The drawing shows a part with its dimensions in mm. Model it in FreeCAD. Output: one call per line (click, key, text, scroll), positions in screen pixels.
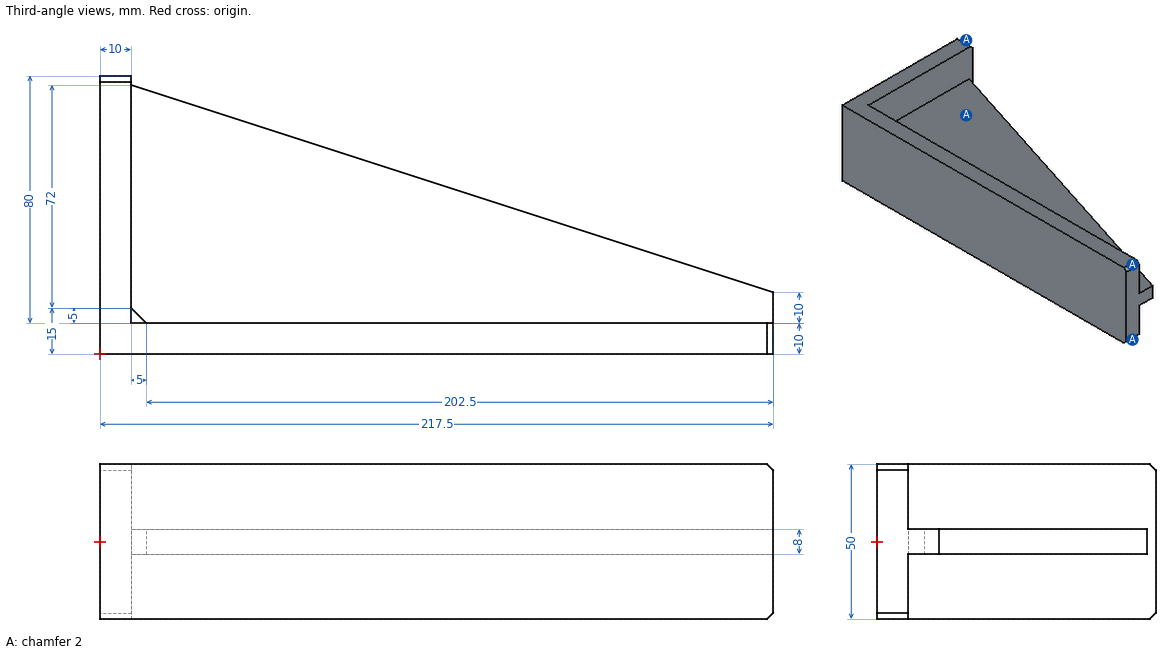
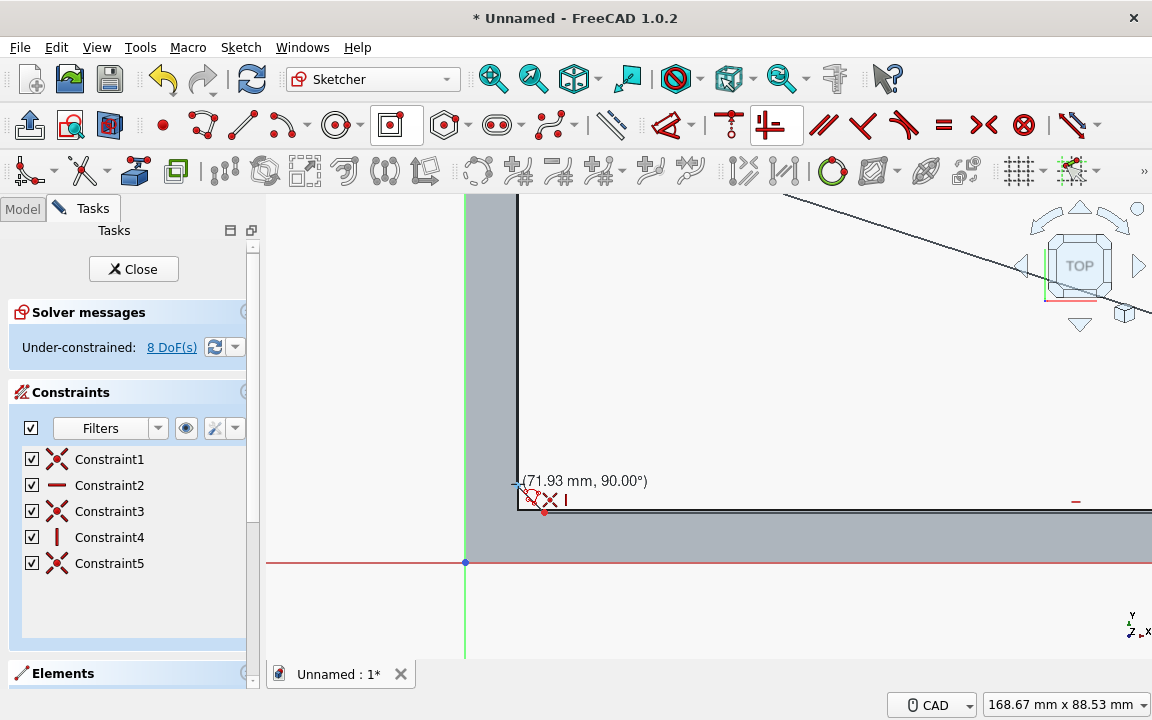
click(518, 486)
key(Escape)
key(Escape)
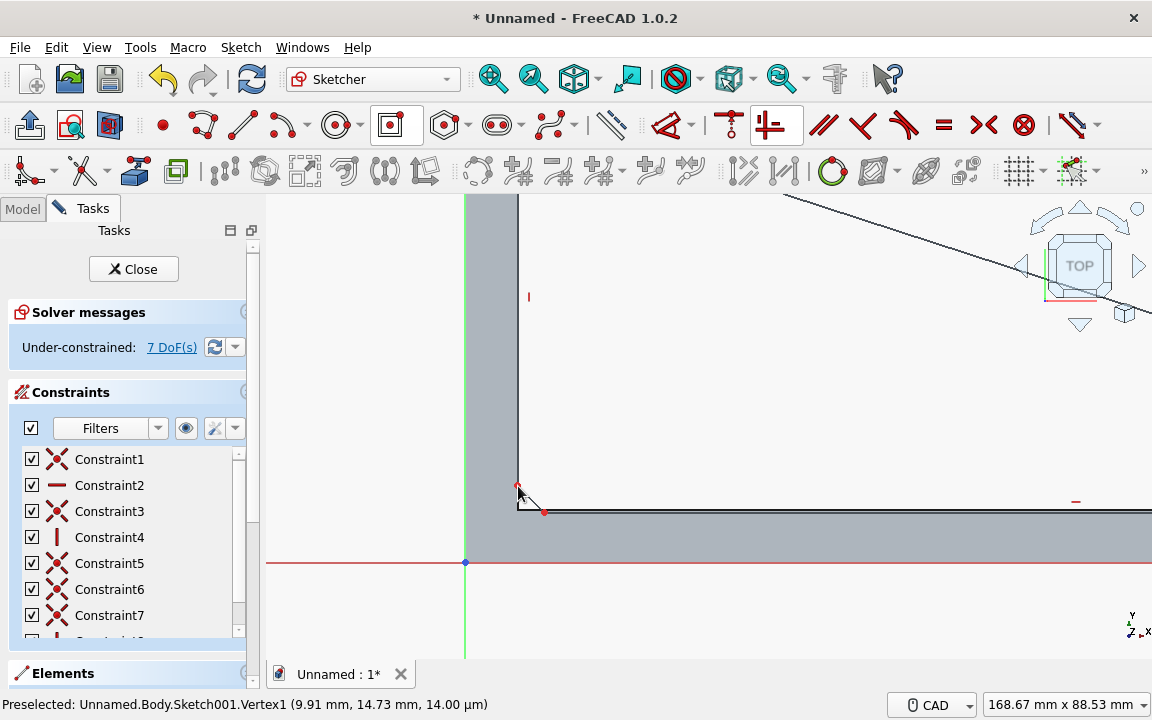
click(666, 126)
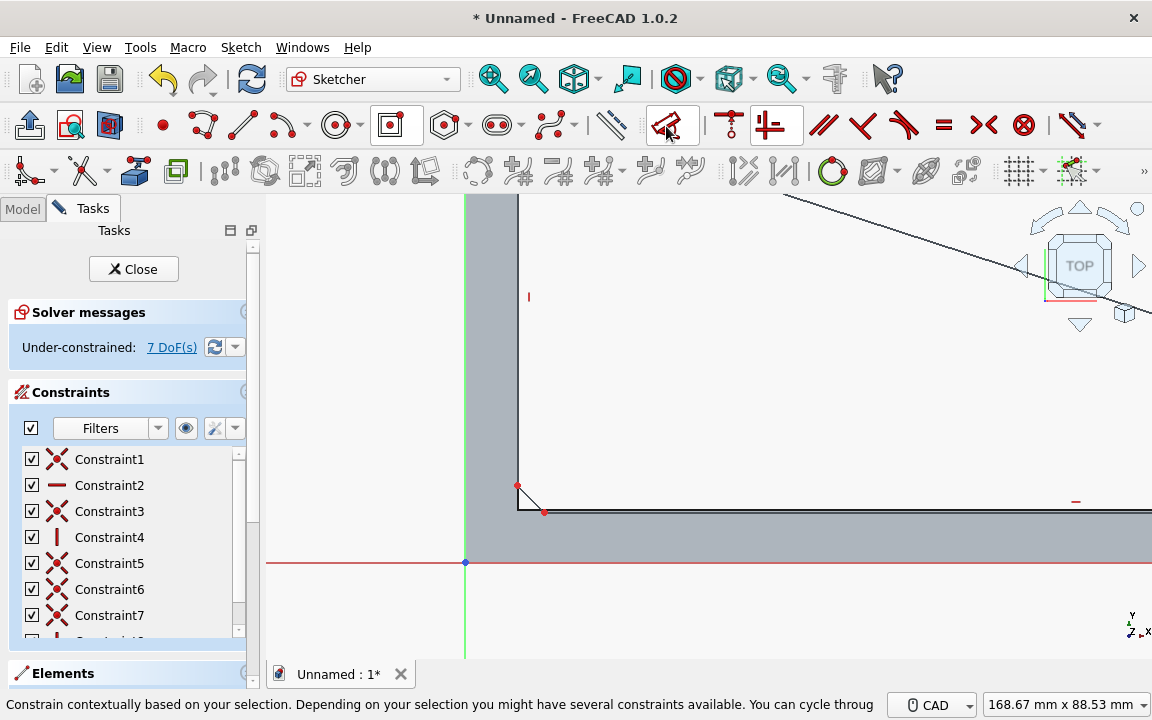
scroll(317, 502, down, 4)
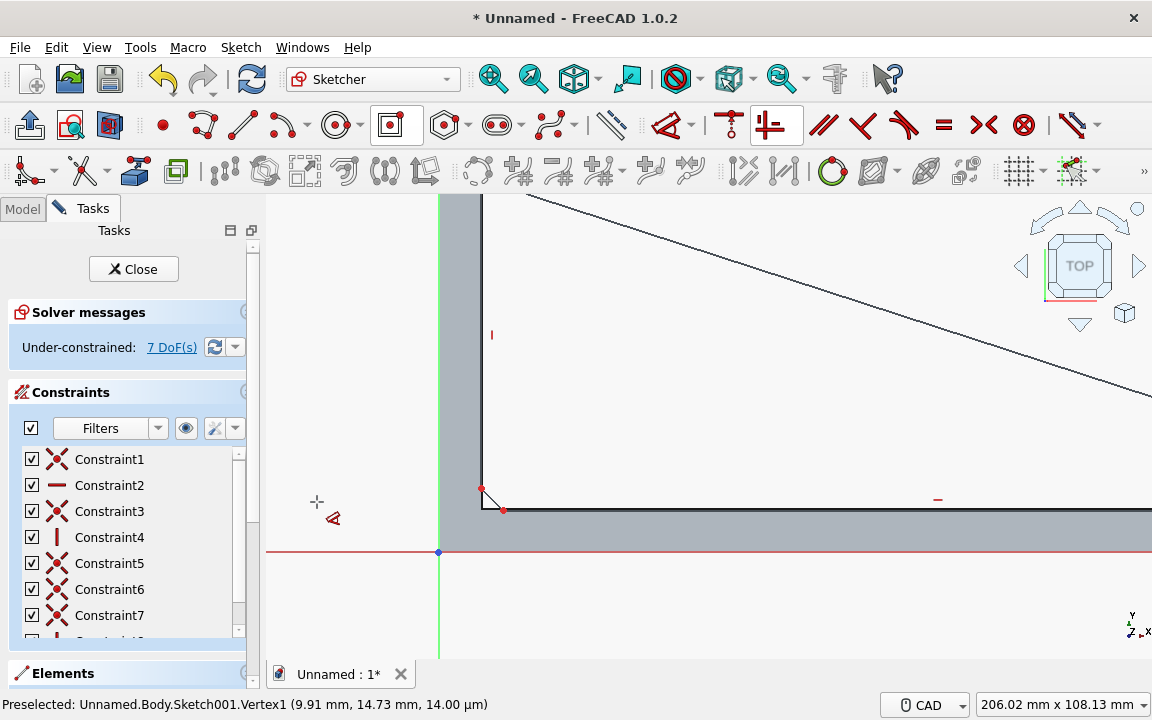
scroll(897, 500, up, 4)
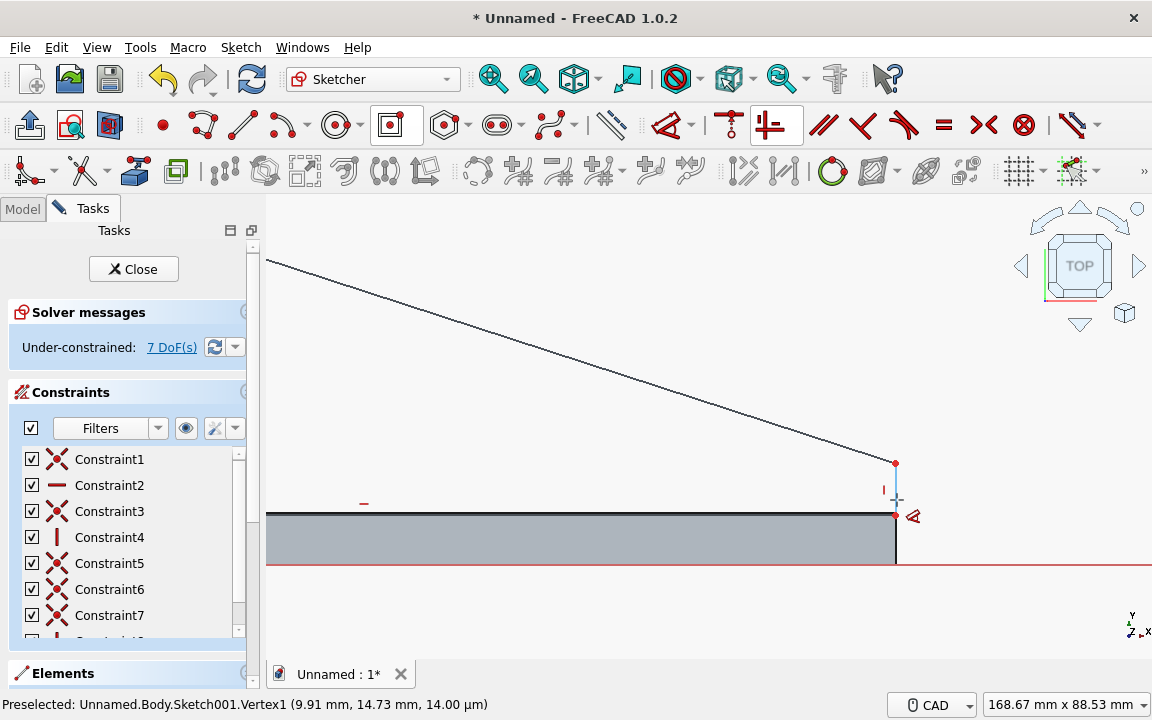
click(896, 500)
click(930, 489)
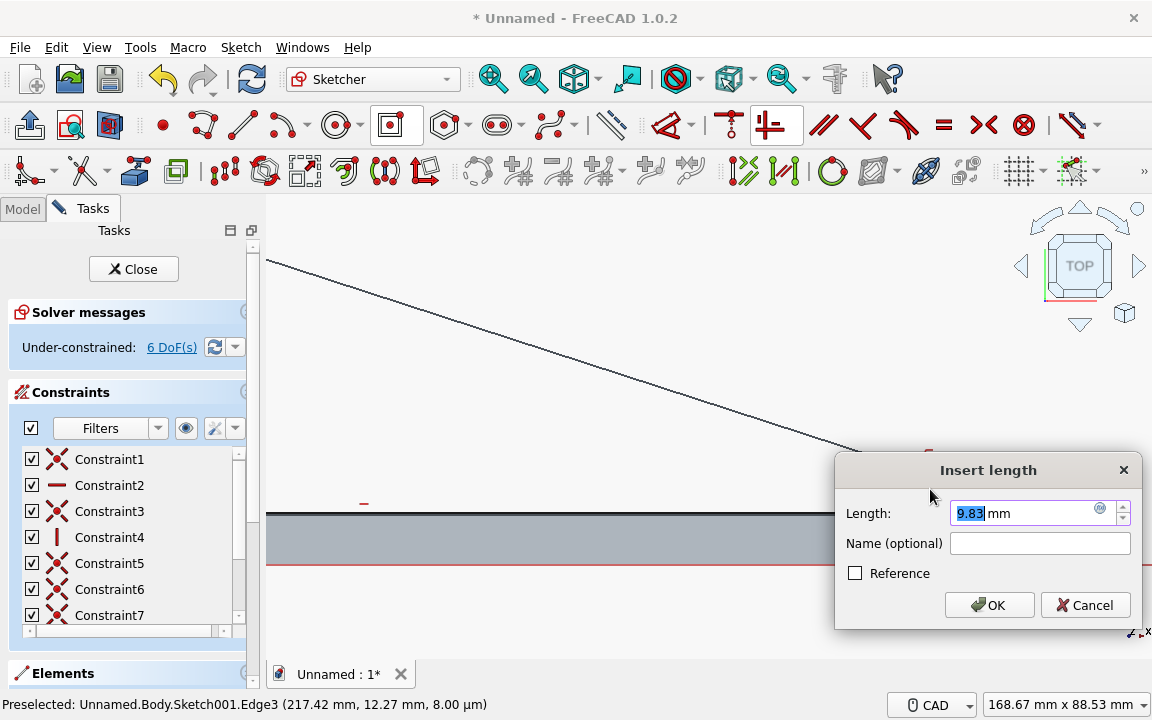
text(10)
key(Return)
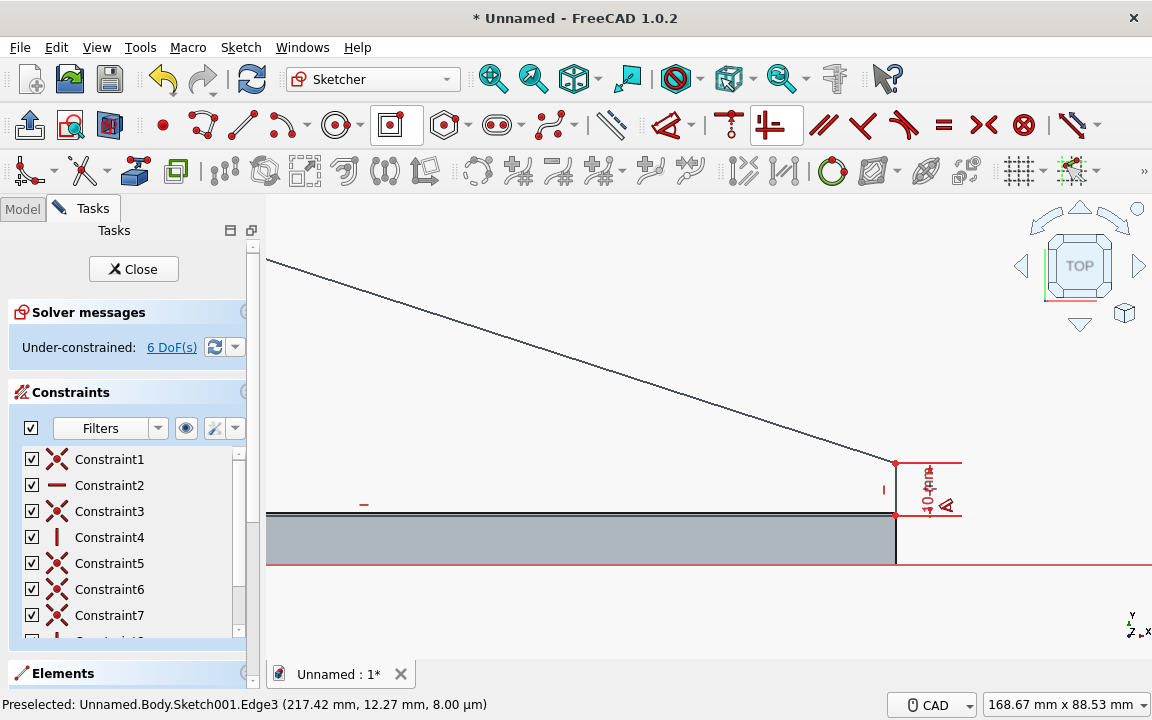
scroll(898, 500, down, 4)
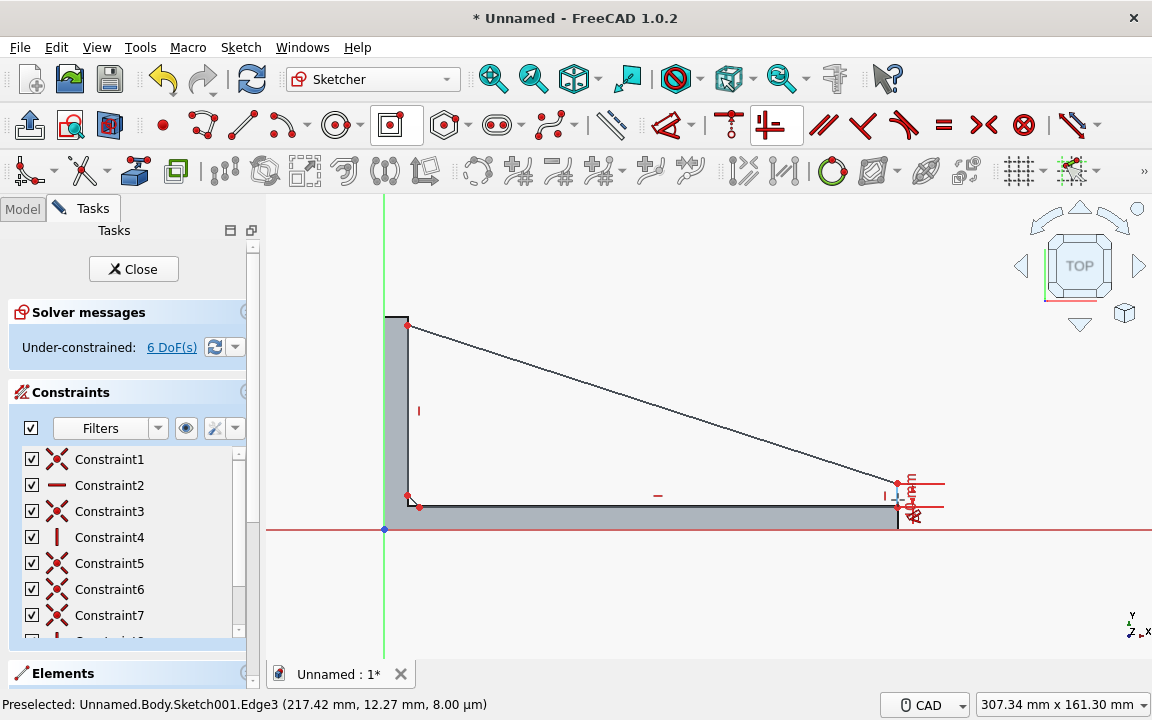
click(408, 376)
click(442, 410)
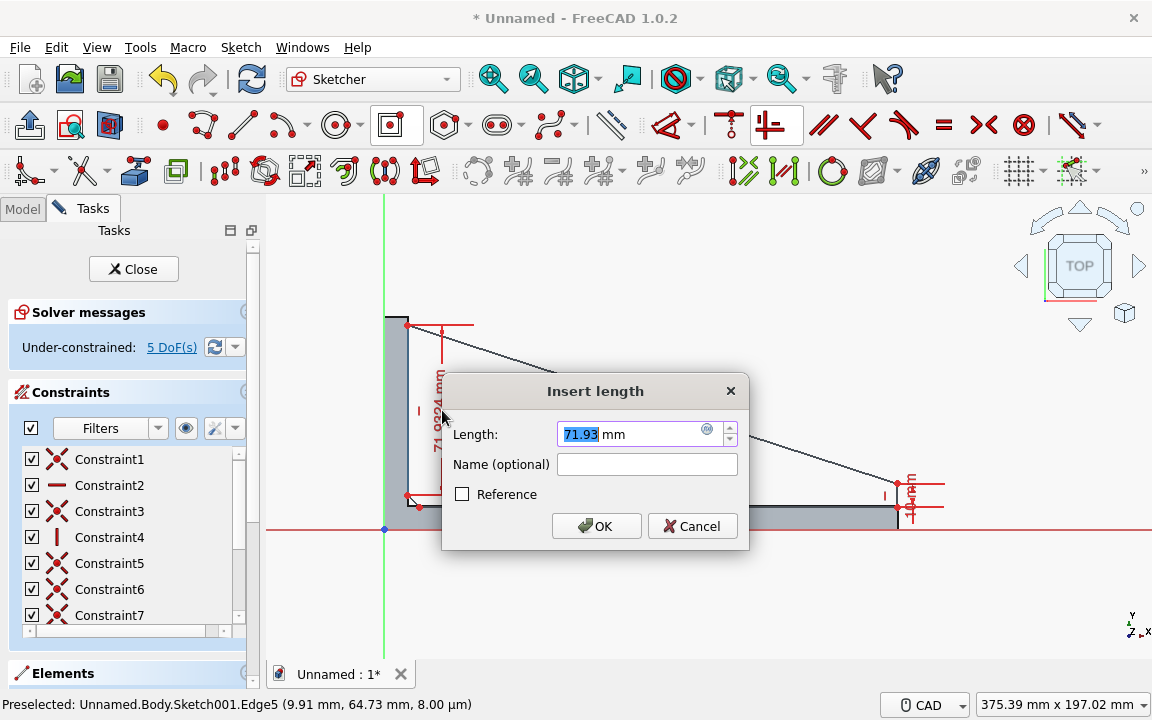
text(72)
key(Return)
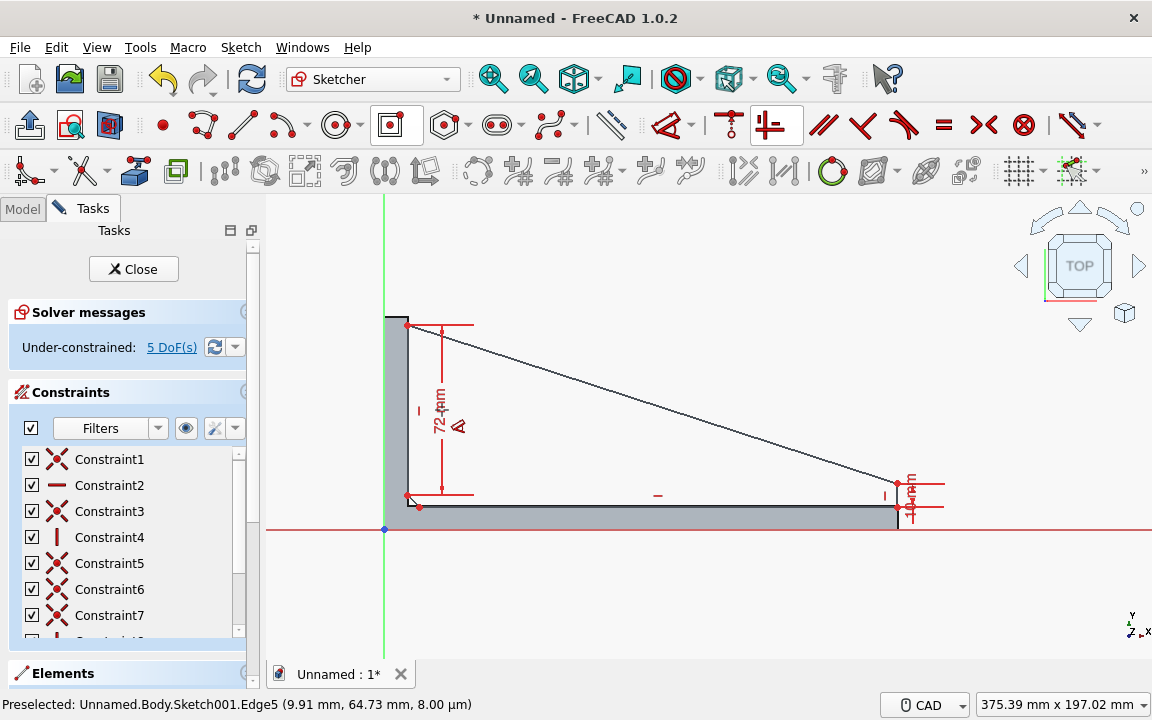
scroll(414, 501, up, 7)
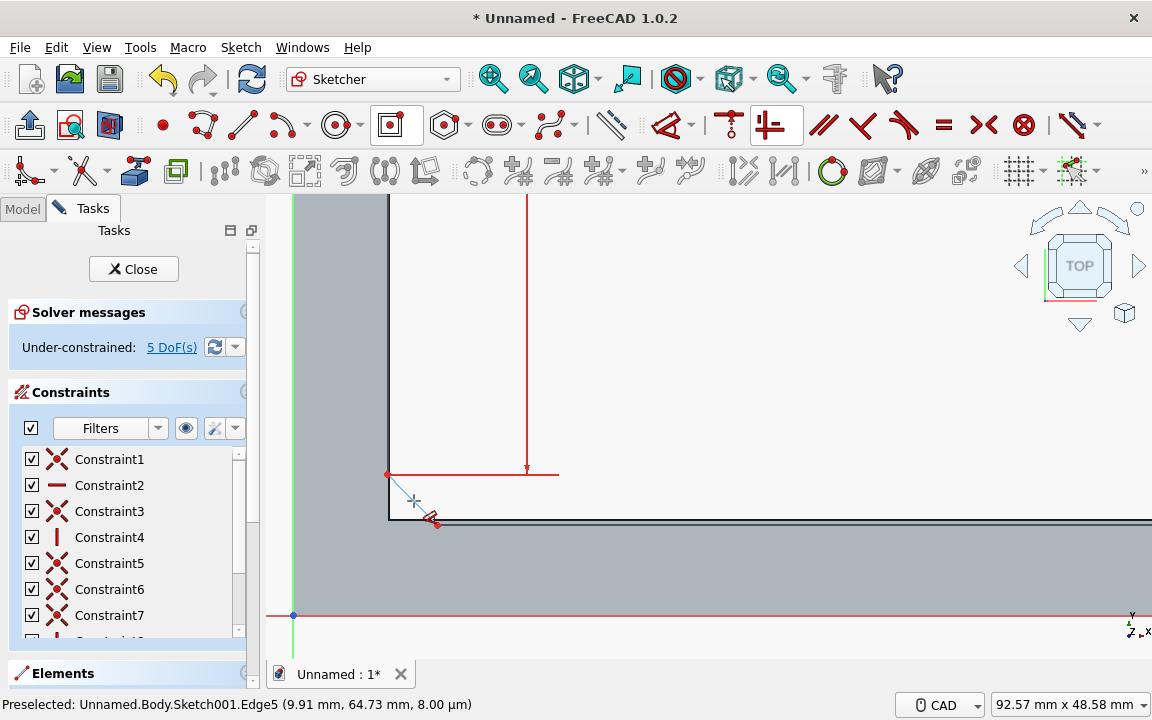
click(413, 500)
click(413, 559)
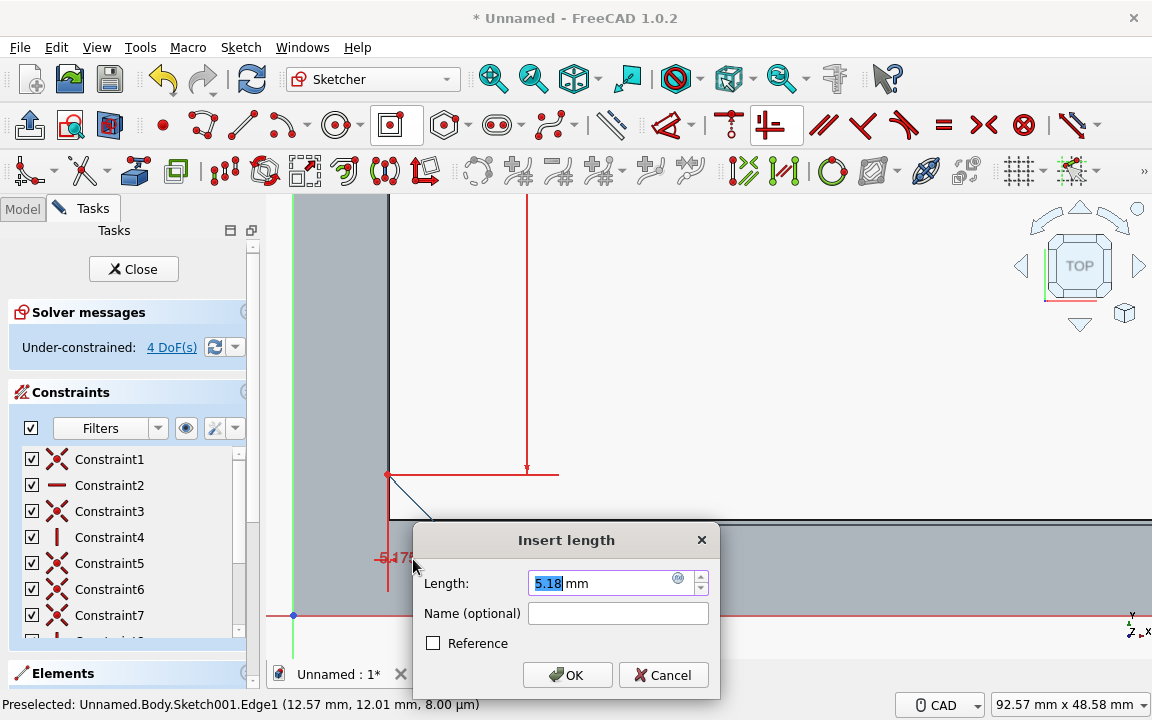
text(5)
key(Return)